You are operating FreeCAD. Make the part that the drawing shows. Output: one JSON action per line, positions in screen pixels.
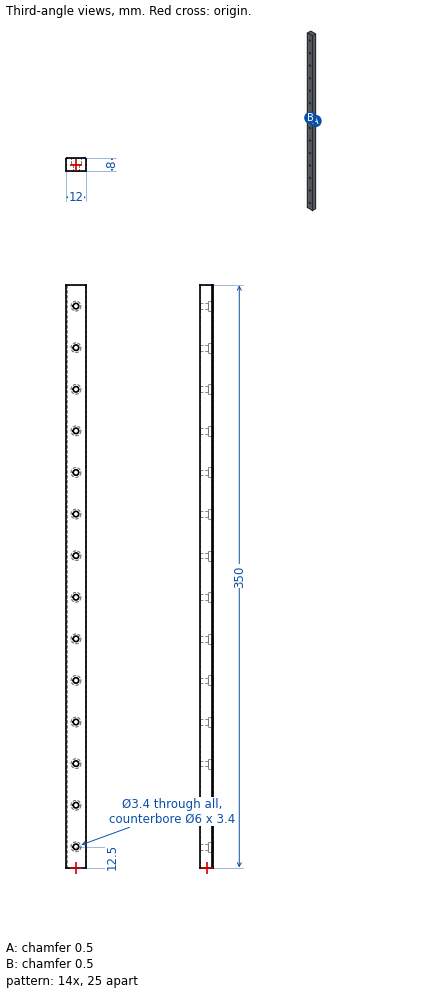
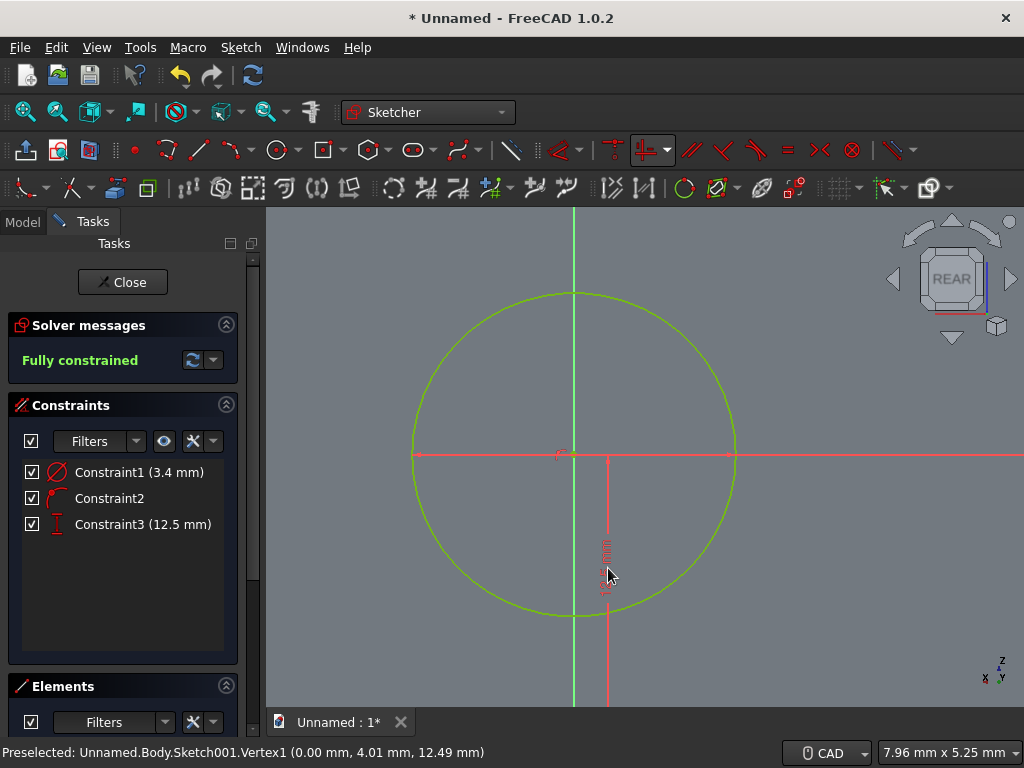
{"action": "left_click", "coordinate": [123, 282]}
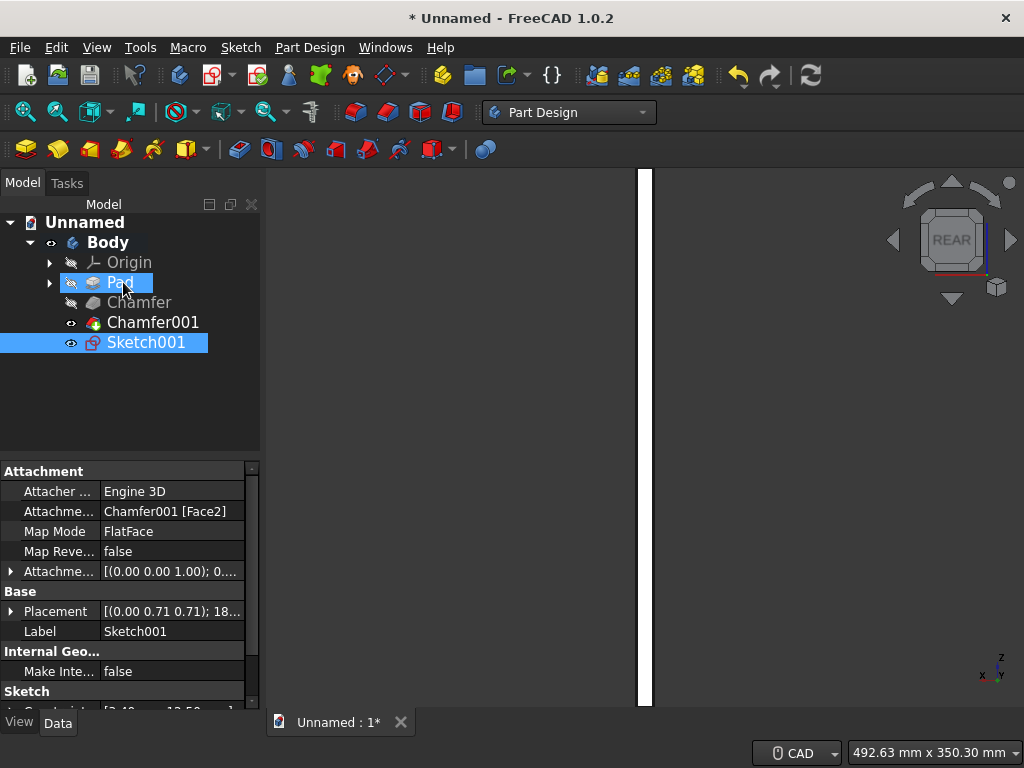
{"action": "left_click", "coordinate": [272, 150]}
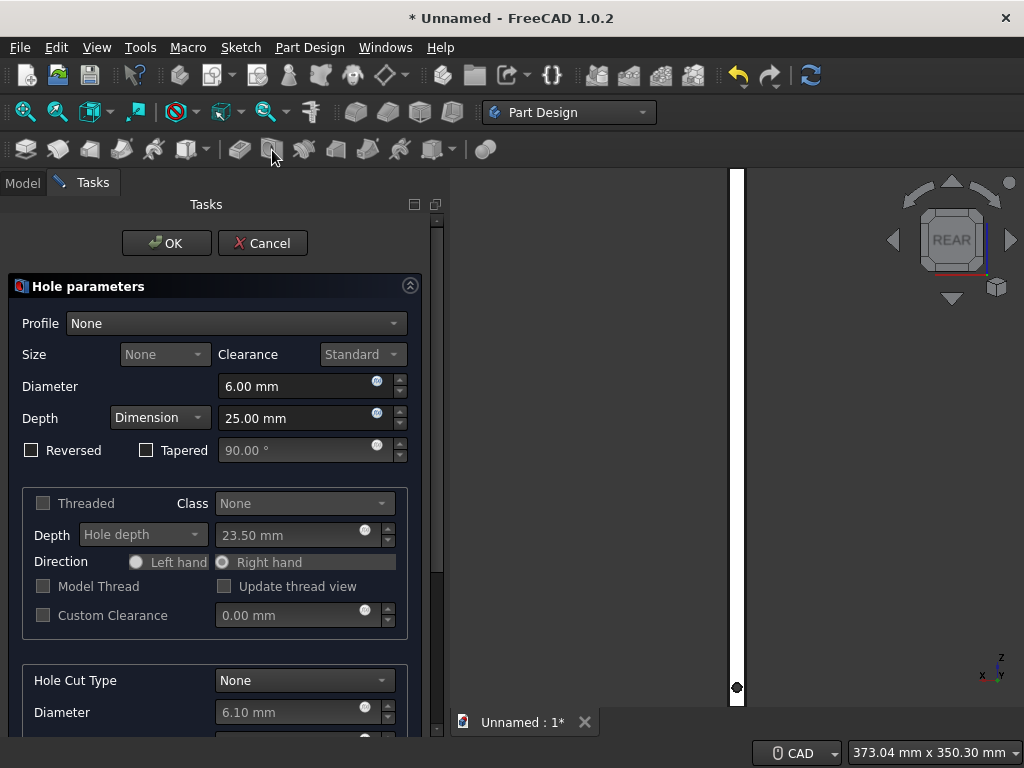
{"action": "triple_click", "coordinate": [305, 386]}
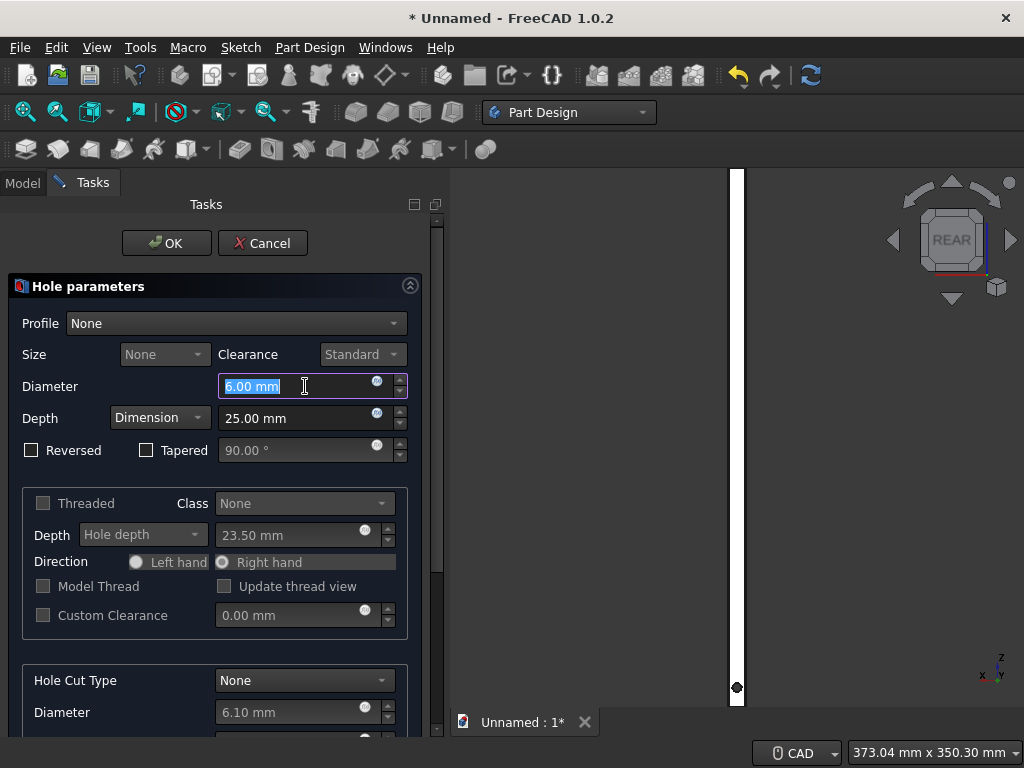
{"action": "type", "text": "3.4"}
{"action": "key", "text": "Tab"}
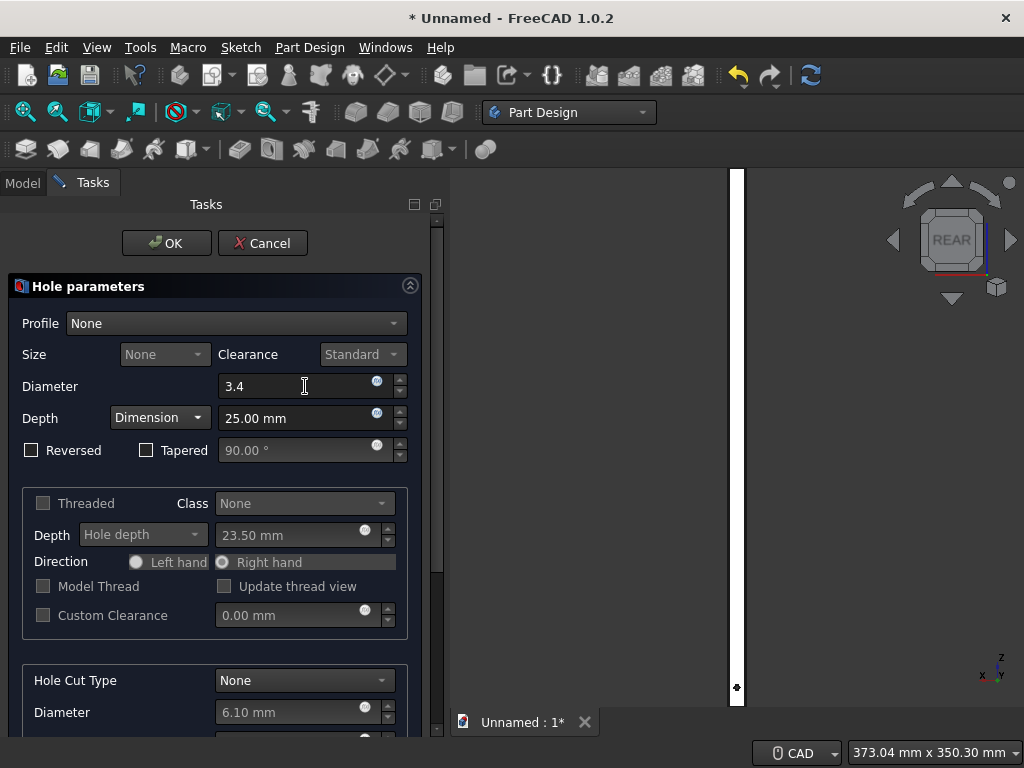
{"action": "left_click", "coordinate": [161, 418]}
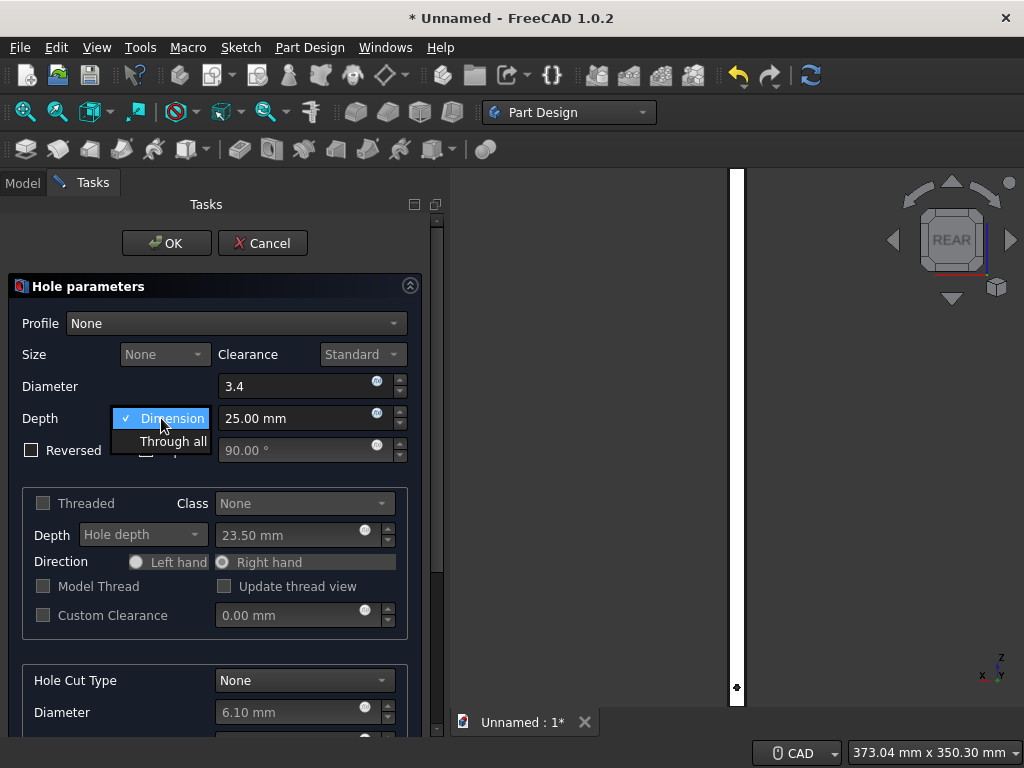
{"action": "left_click", "coordinate": [160, 442]}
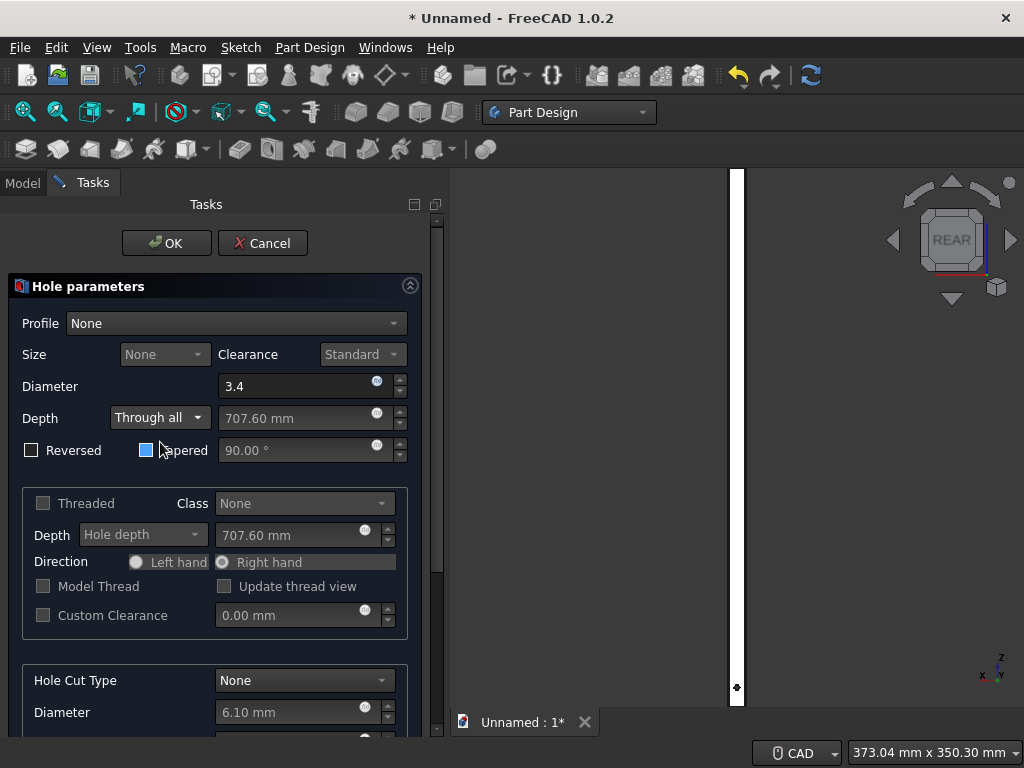
{"action": "left_click", "coordinate": [306, 680]}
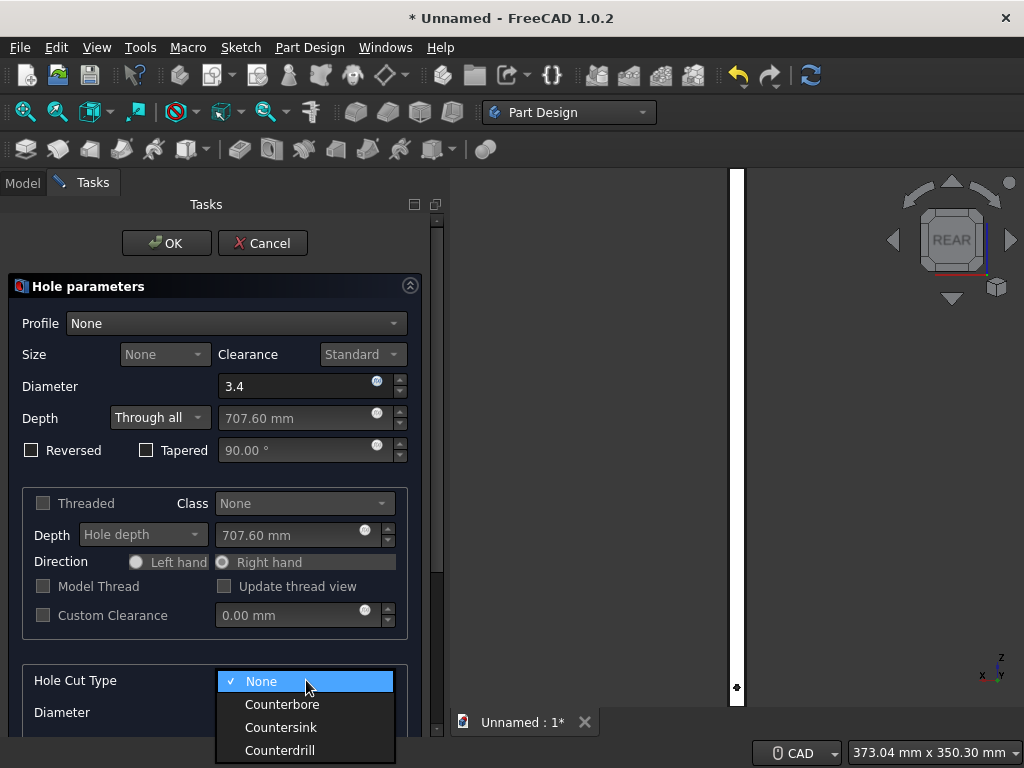
{"action": "left_click", "coordinate": [304, 704]}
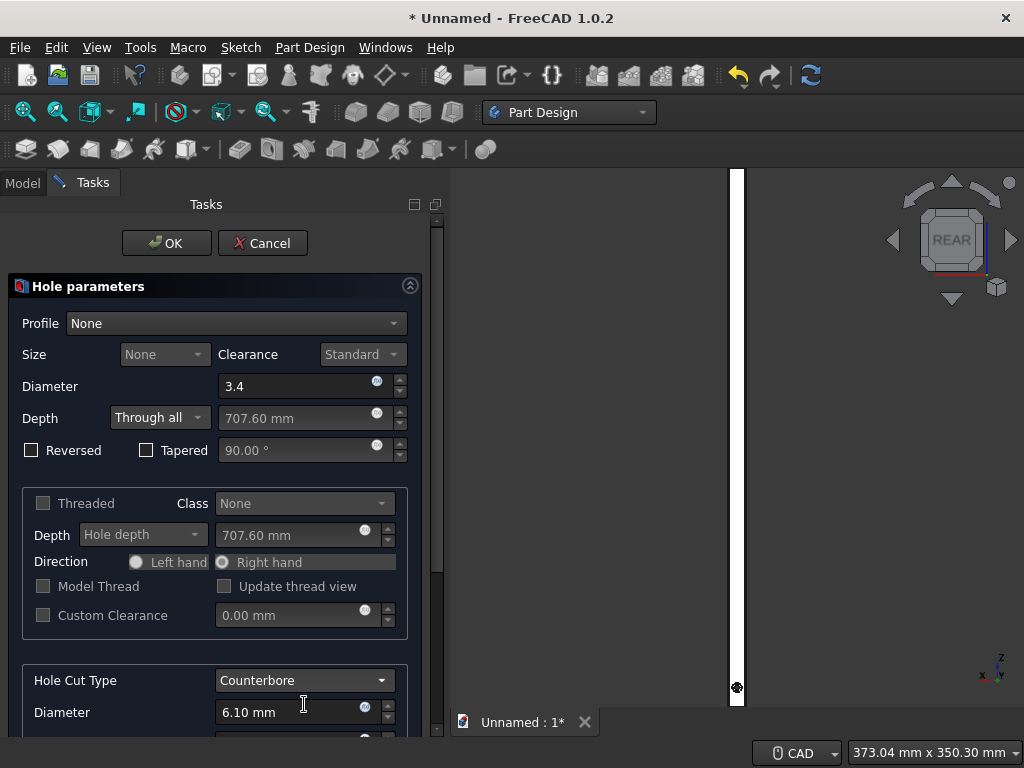
{"action": "triple_click", "coordinate": [298, 712]}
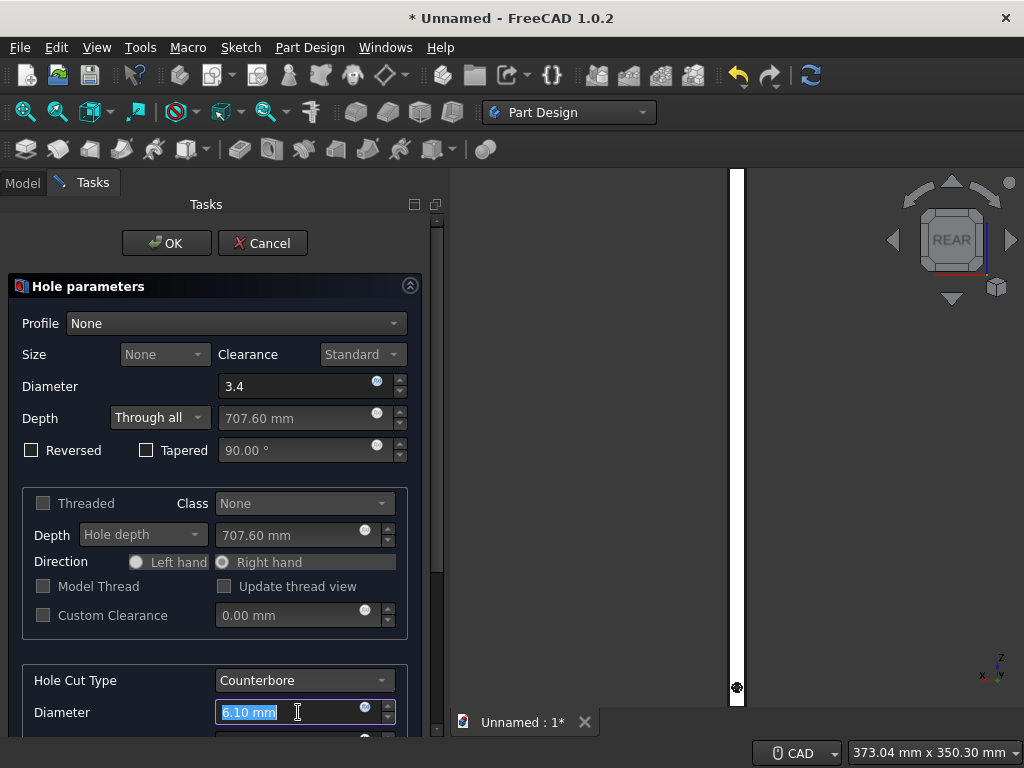
{"action": "type", "text": "6"}
{"action": "key", "text": "Tab"}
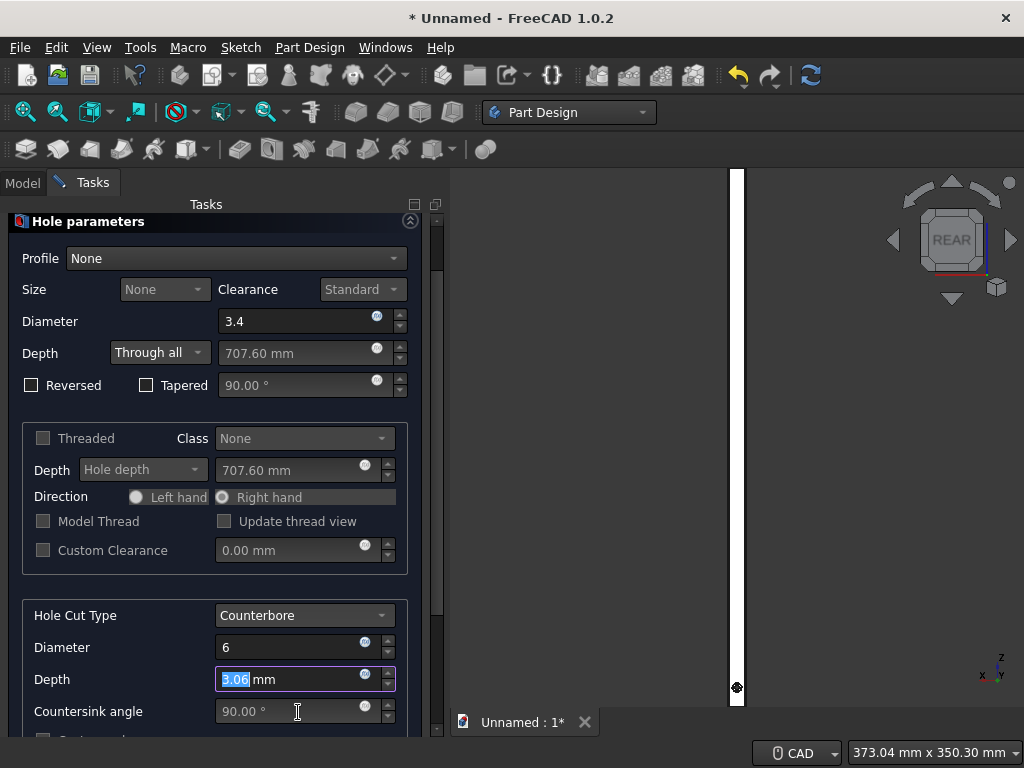
{"action": "type", "text": "3.4"}
{"action": "key", "text": "Tab"}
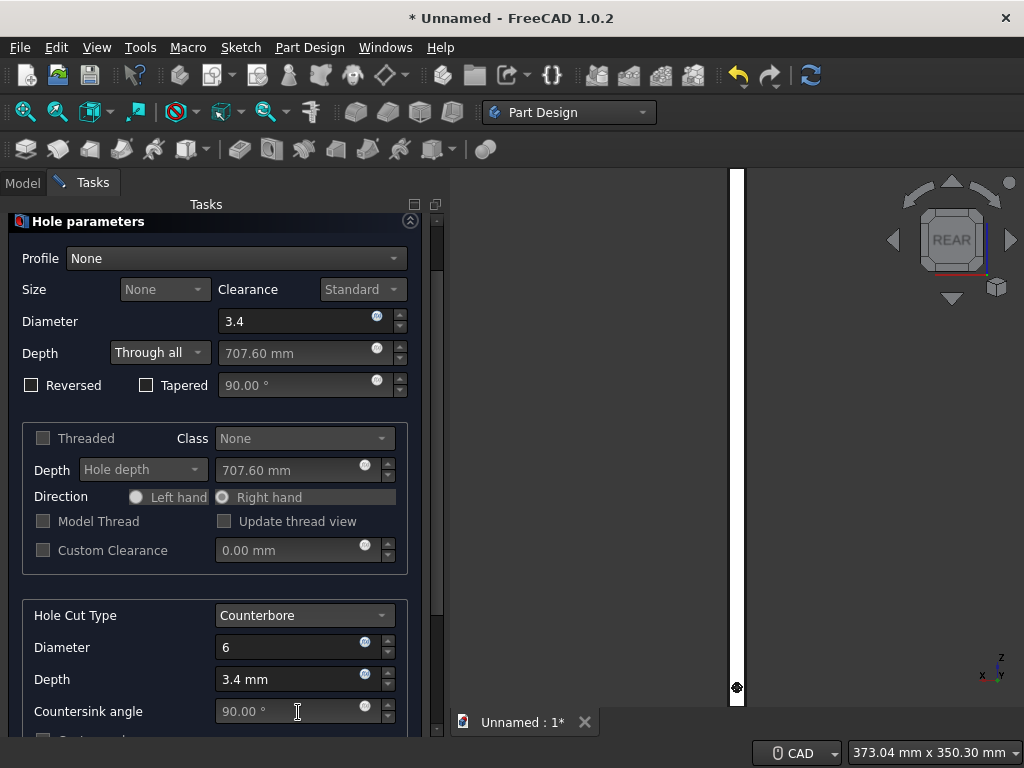
{"action": "scroll", "coordinate": [437, 475], "scroll_direction": "up", "scroll_amount": 2}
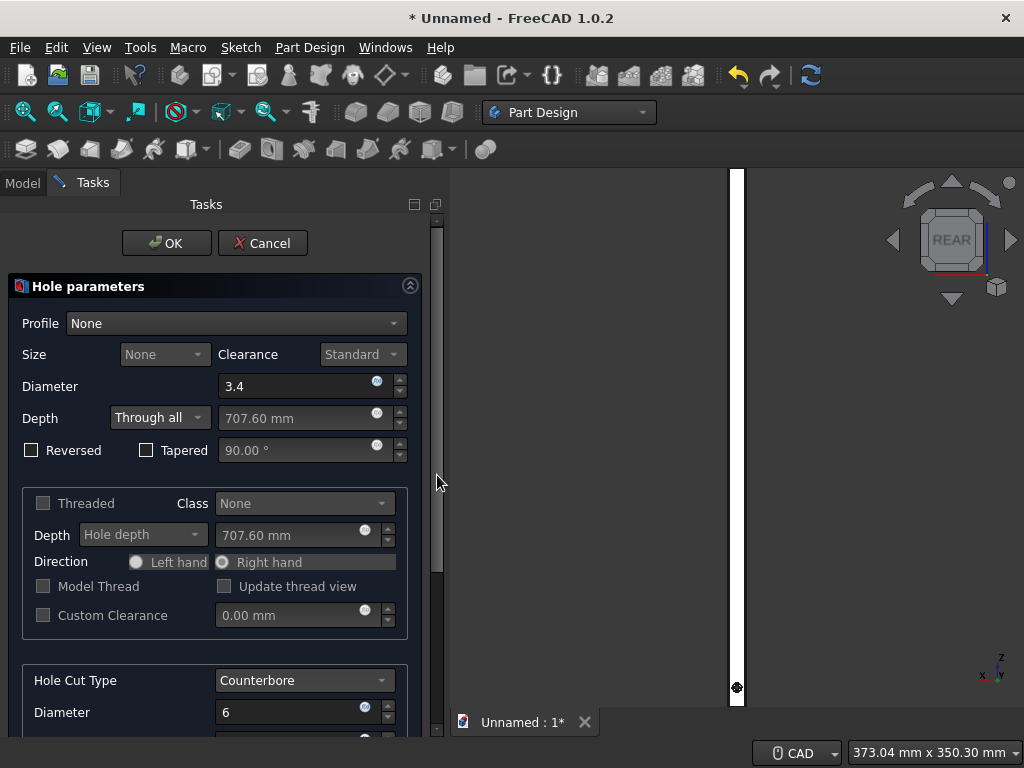
{"action": "left_click", "coordinate": [167, 243]}